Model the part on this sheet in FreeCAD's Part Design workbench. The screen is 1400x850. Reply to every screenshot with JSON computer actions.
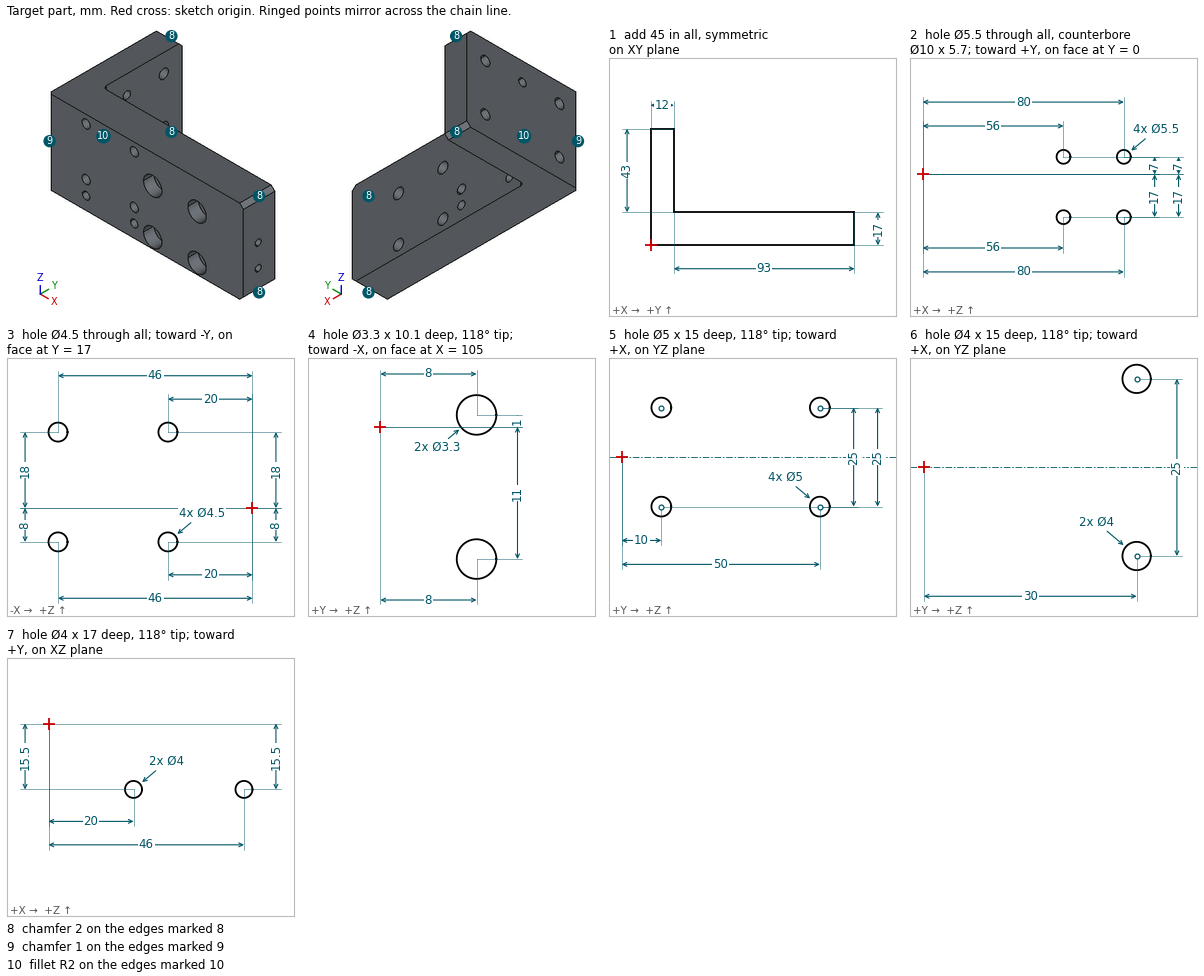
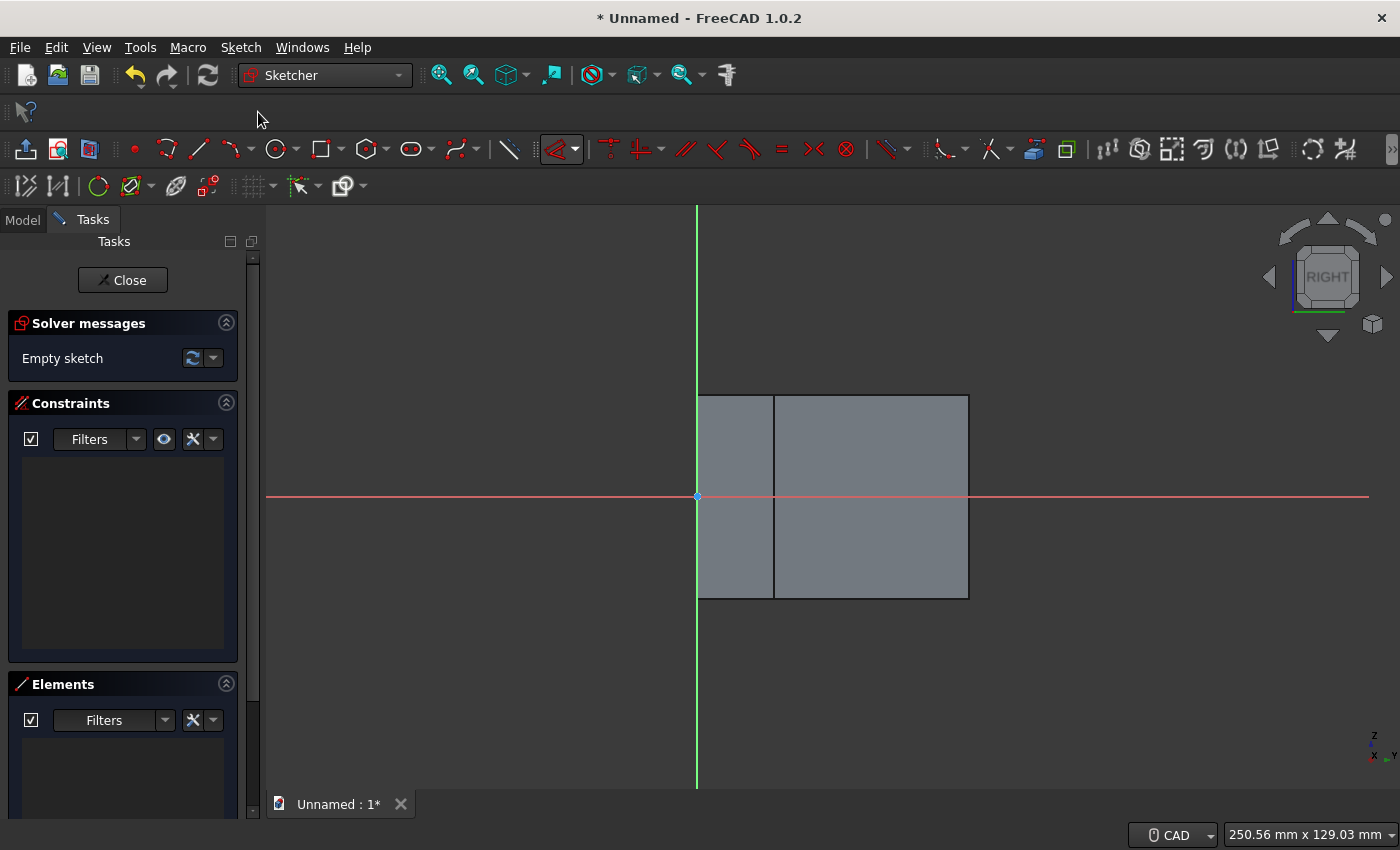
{"action": "scroll", "coordinate": [708, 525], "scroll_direction": "up", "scroll_amount": 8}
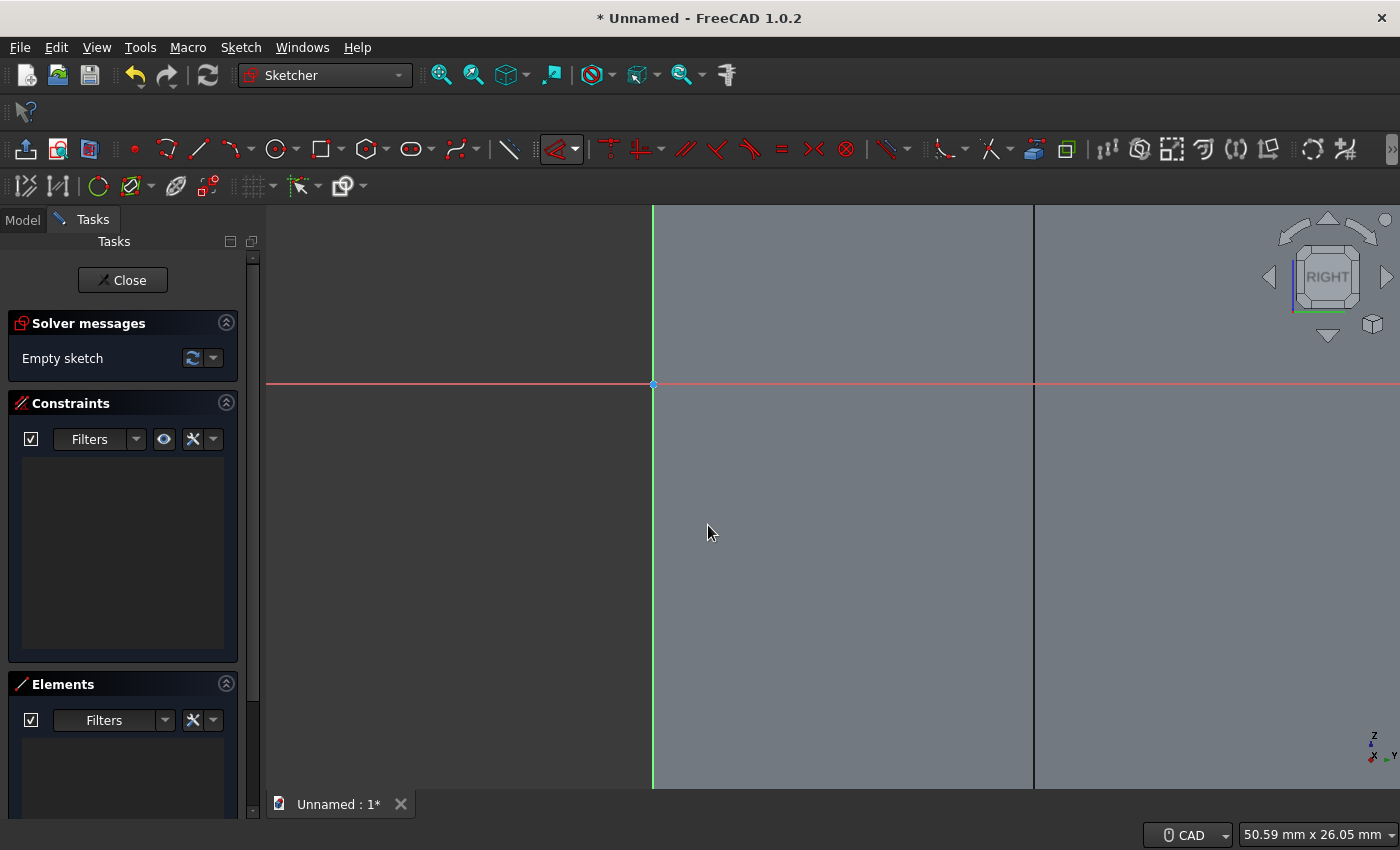
{"action": "key", "text": "g c"}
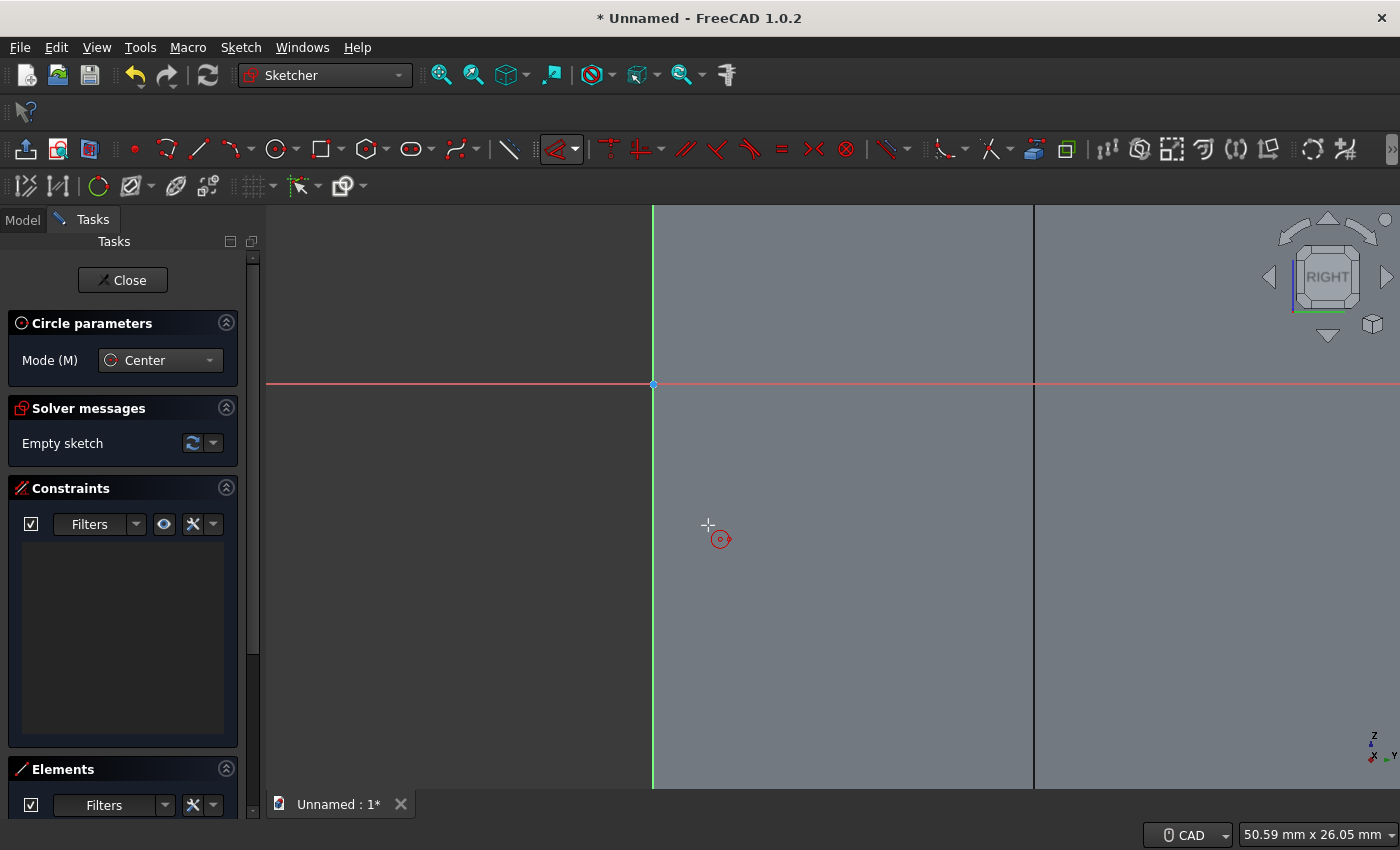
{"action": "left_click", "coordinate": [832, 362]}
{"action": "left_click", "coordinate": [859, 336]}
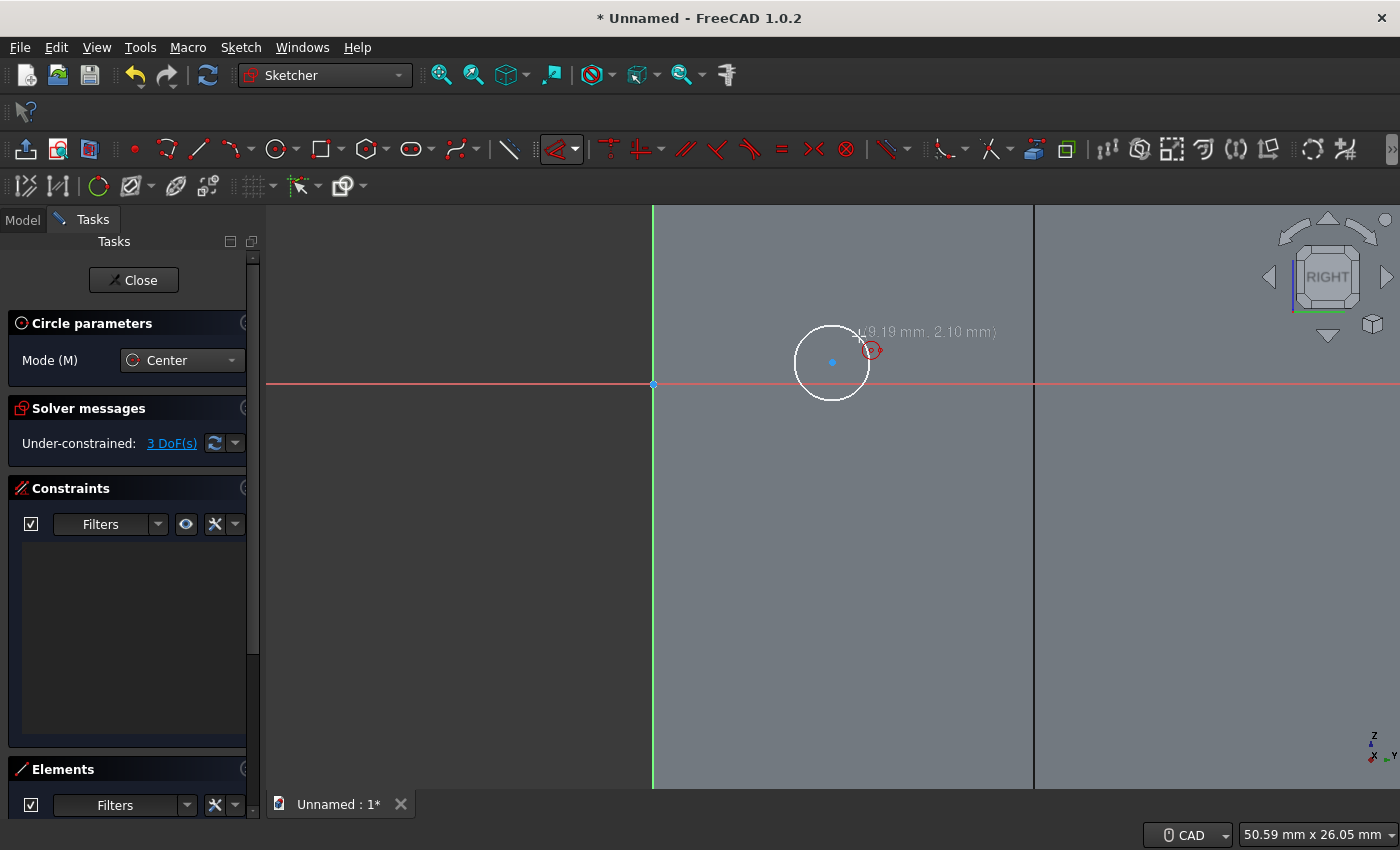
{"action": "left_click", "coordinate": [832, 631]}
{"action": "left_click", "coordinate": [859, 605]}
{"action": "key", "text": "Escape"}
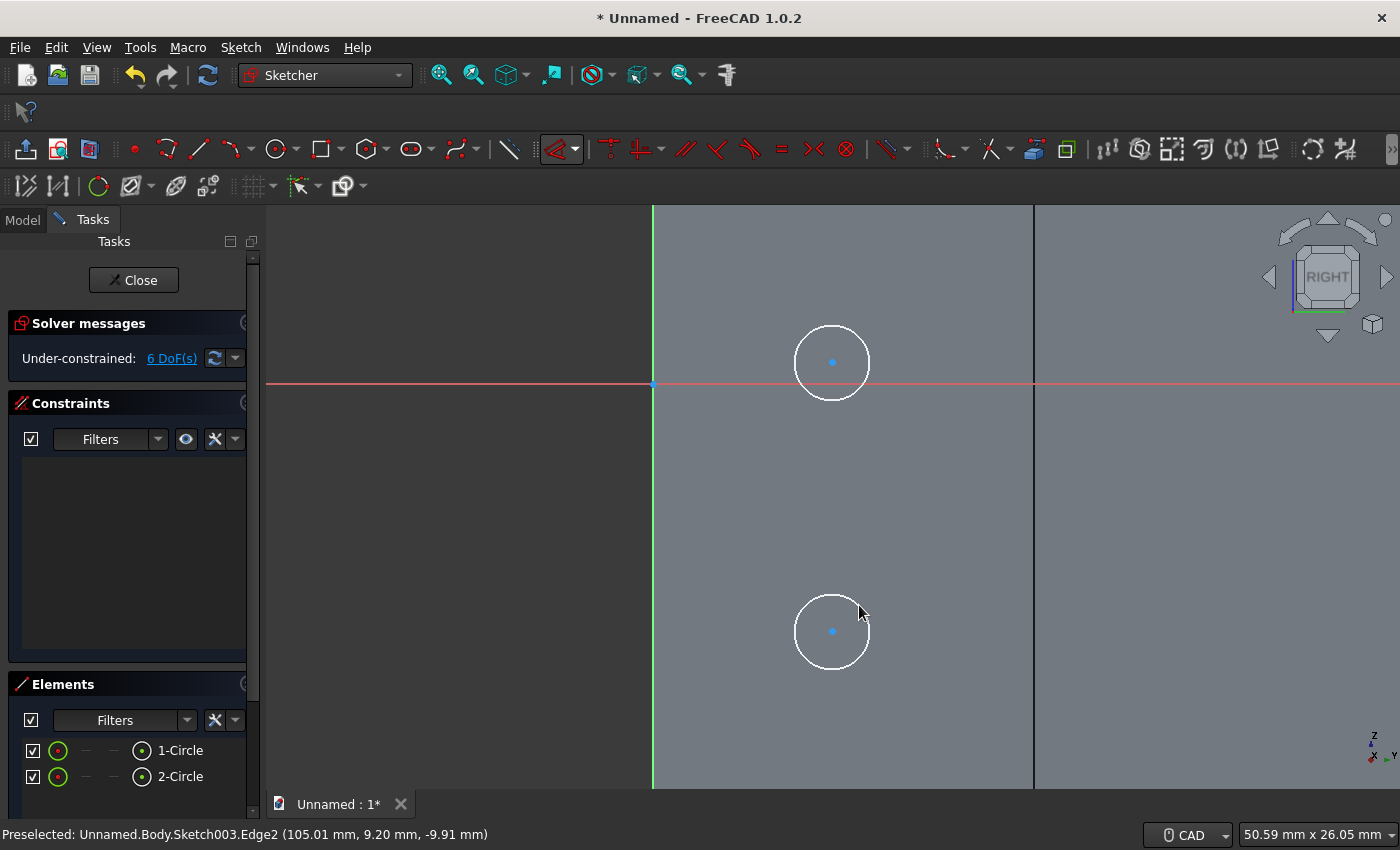
{"action": "left_click", "coordinate": [858, 336]}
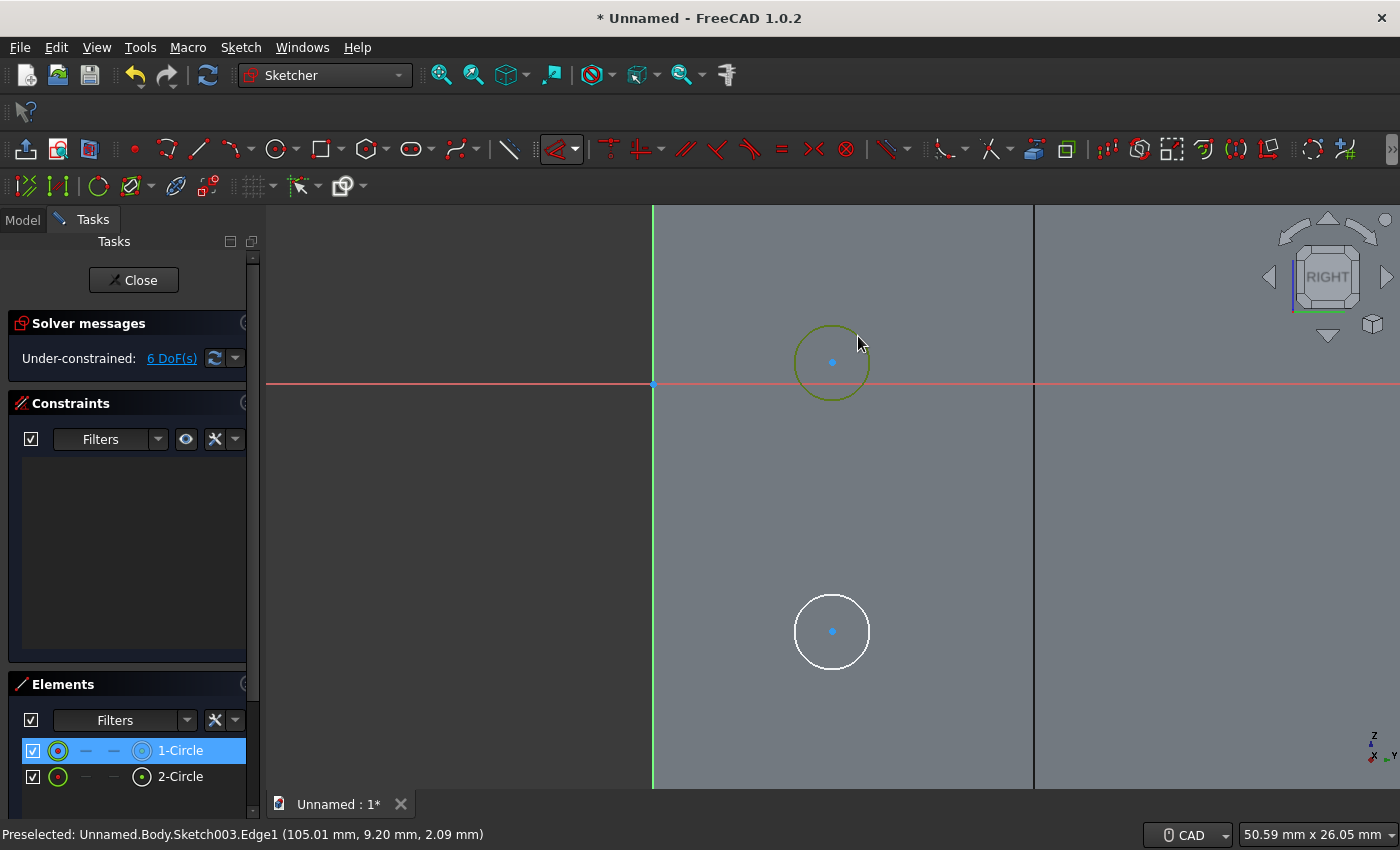
{"action": "left_click", "coordinate": [858, 605]}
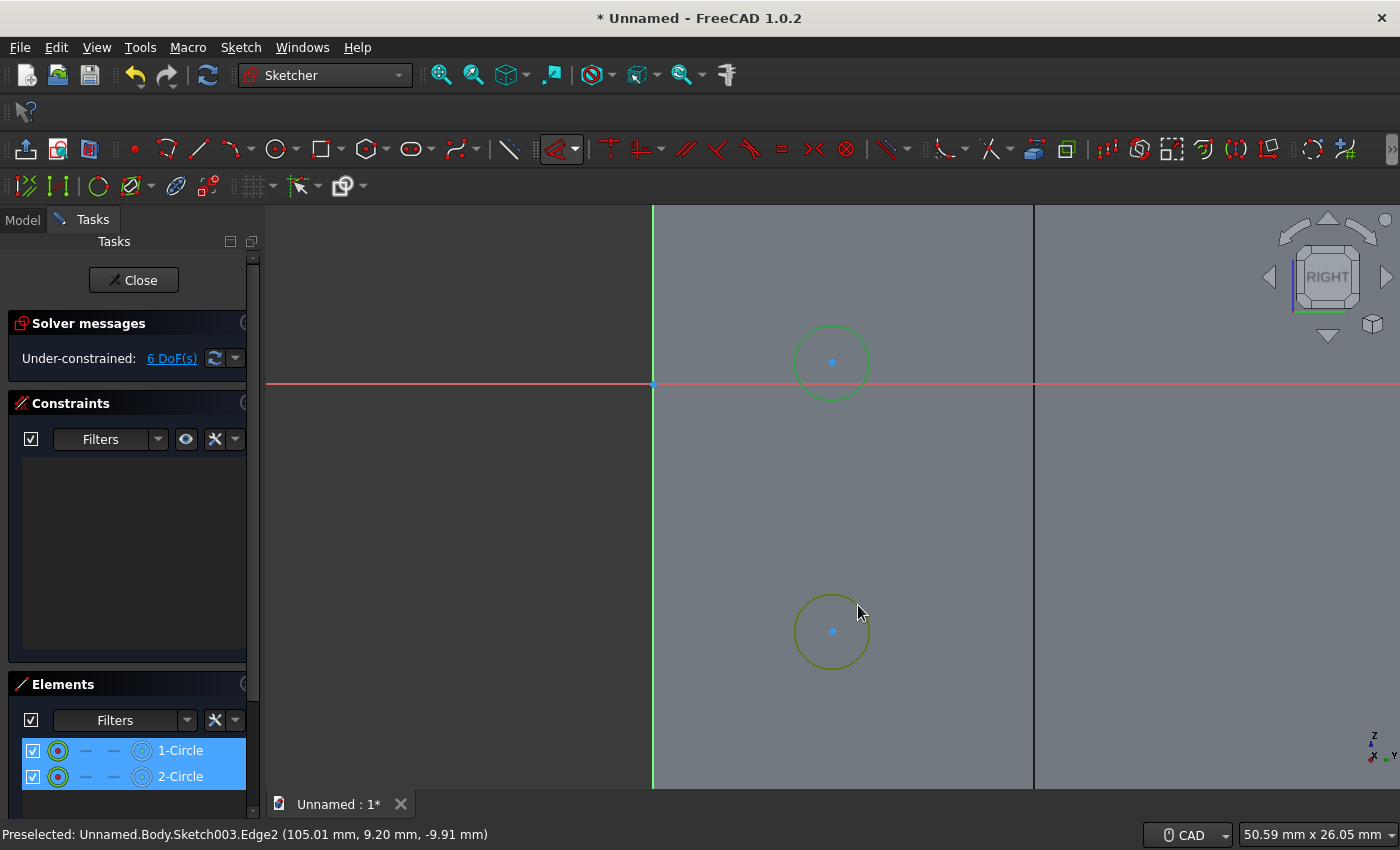
{"action": "key", "text": "e"}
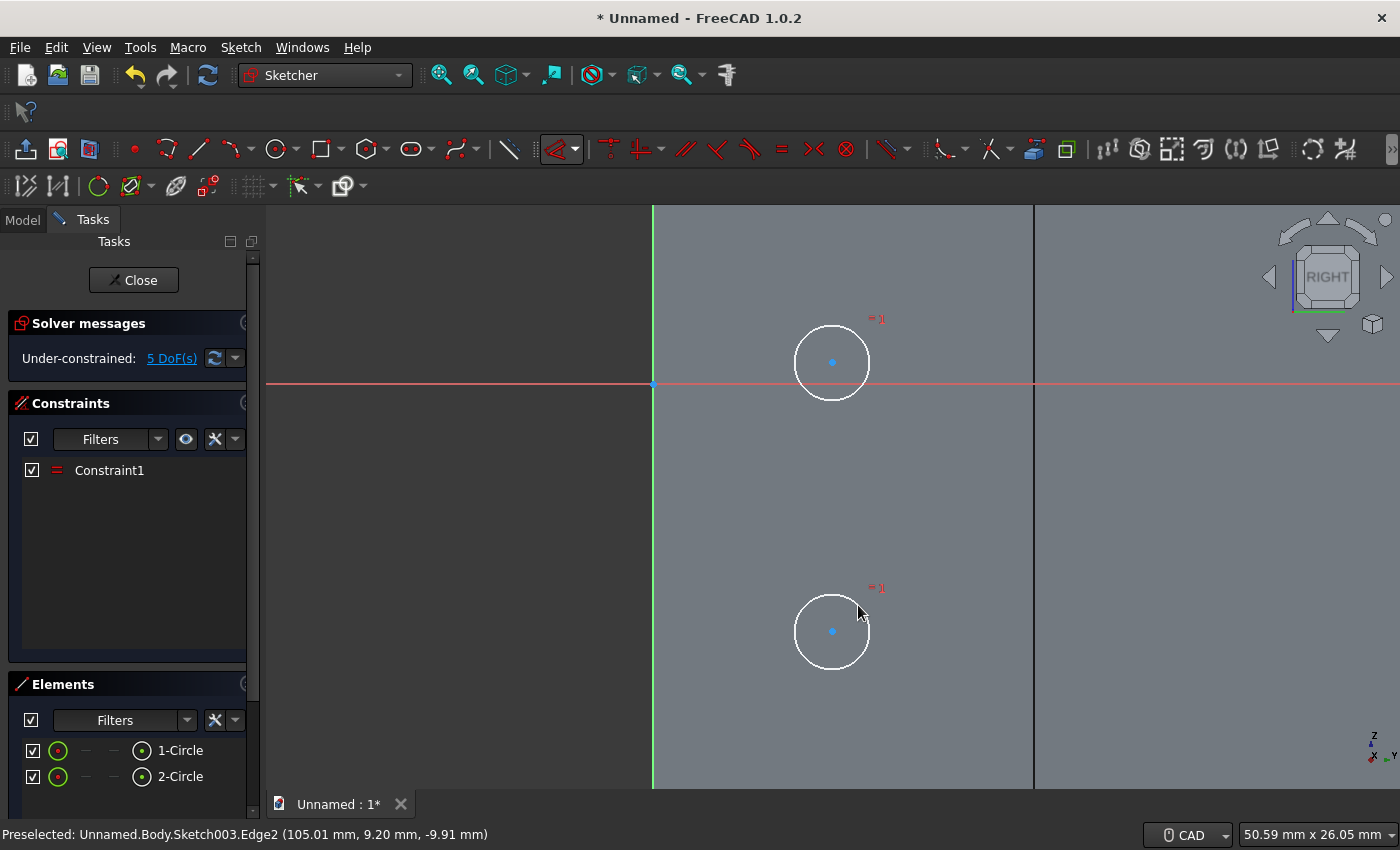
{"action": "left_click", "coordinate": [858, 336]}